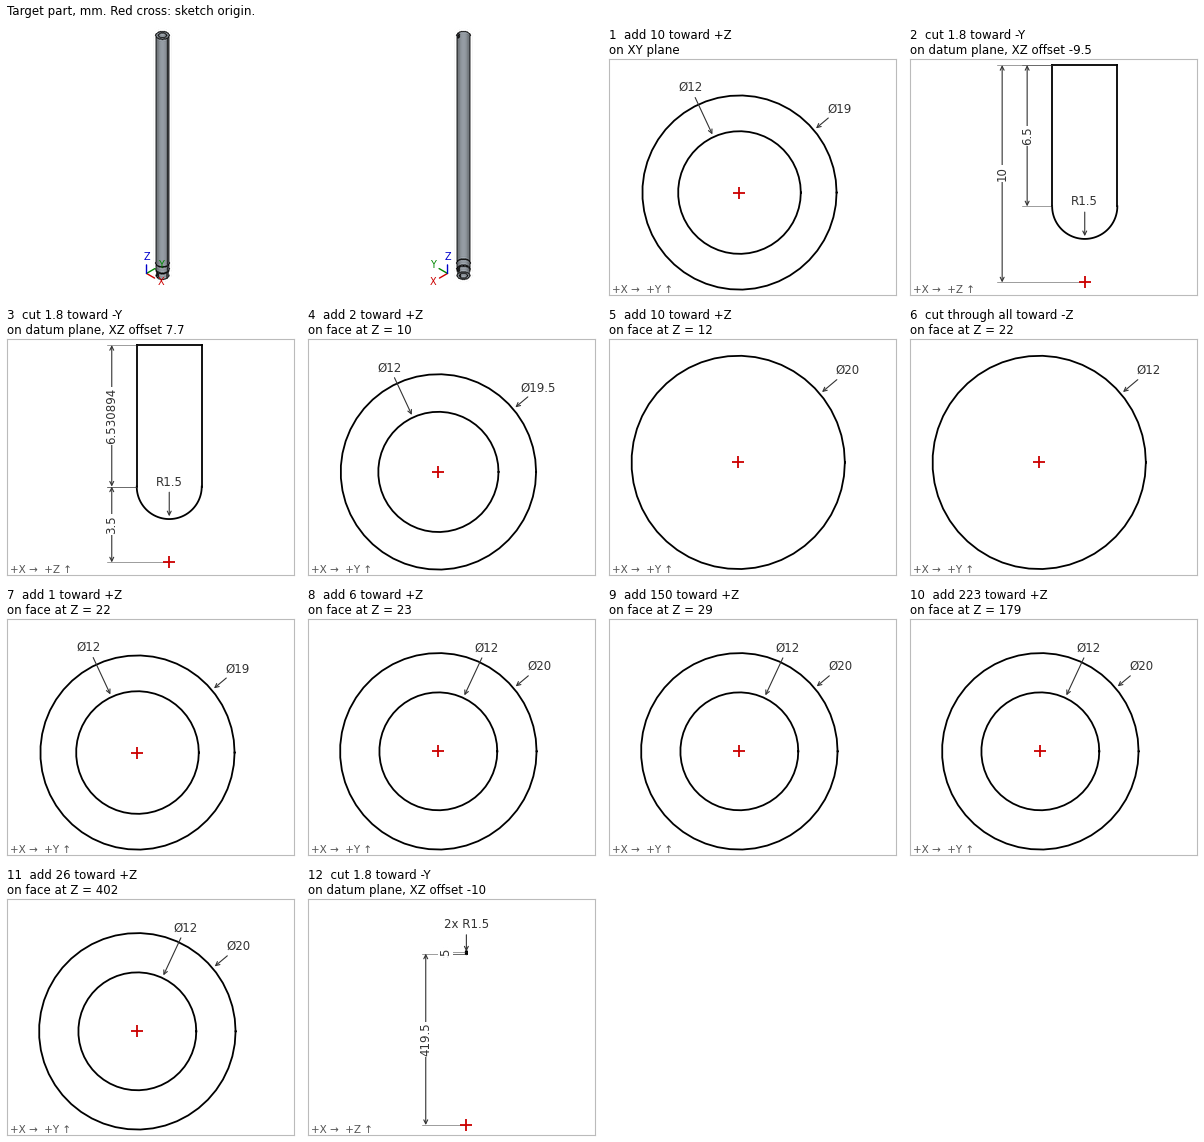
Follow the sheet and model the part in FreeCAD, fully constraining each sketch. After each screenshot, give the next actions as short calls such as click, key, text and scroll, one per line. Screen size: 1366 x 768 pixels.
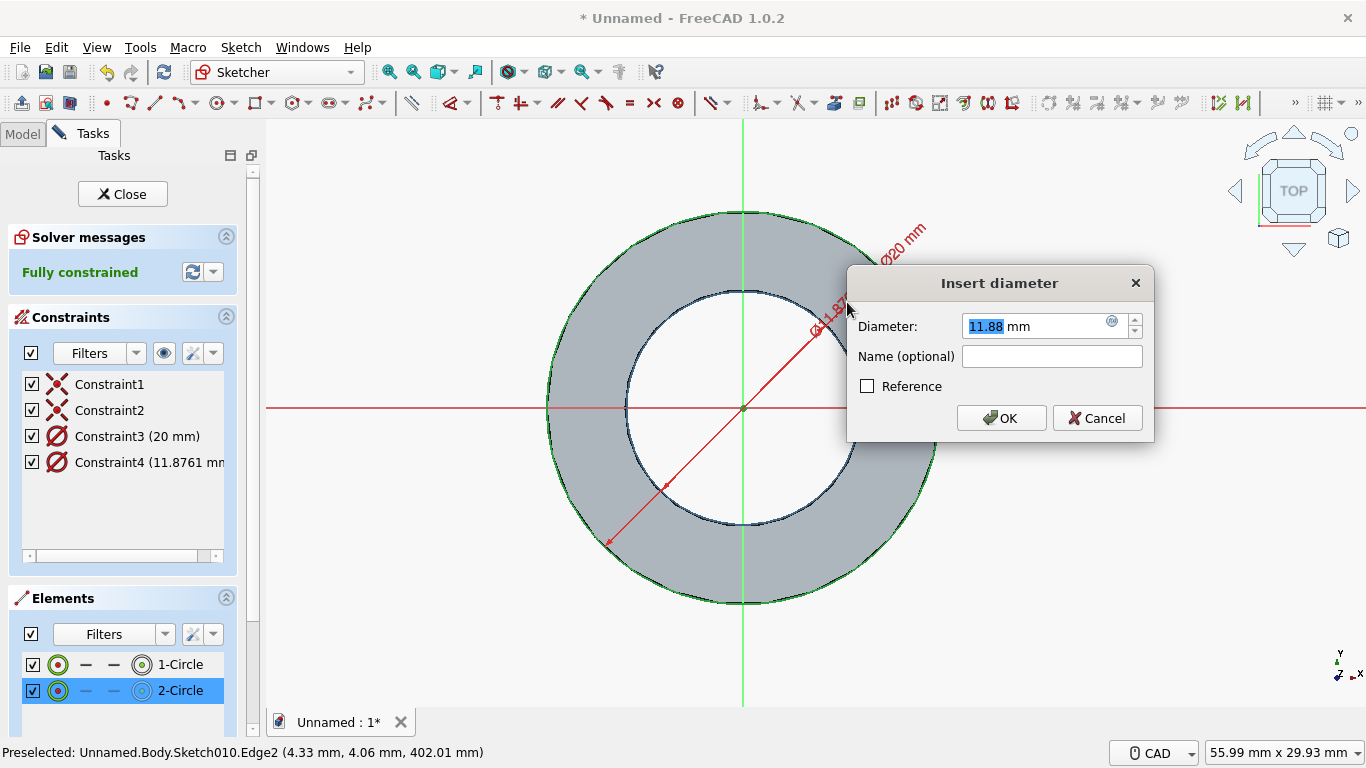
text(12)
key(Return)
key(Escape)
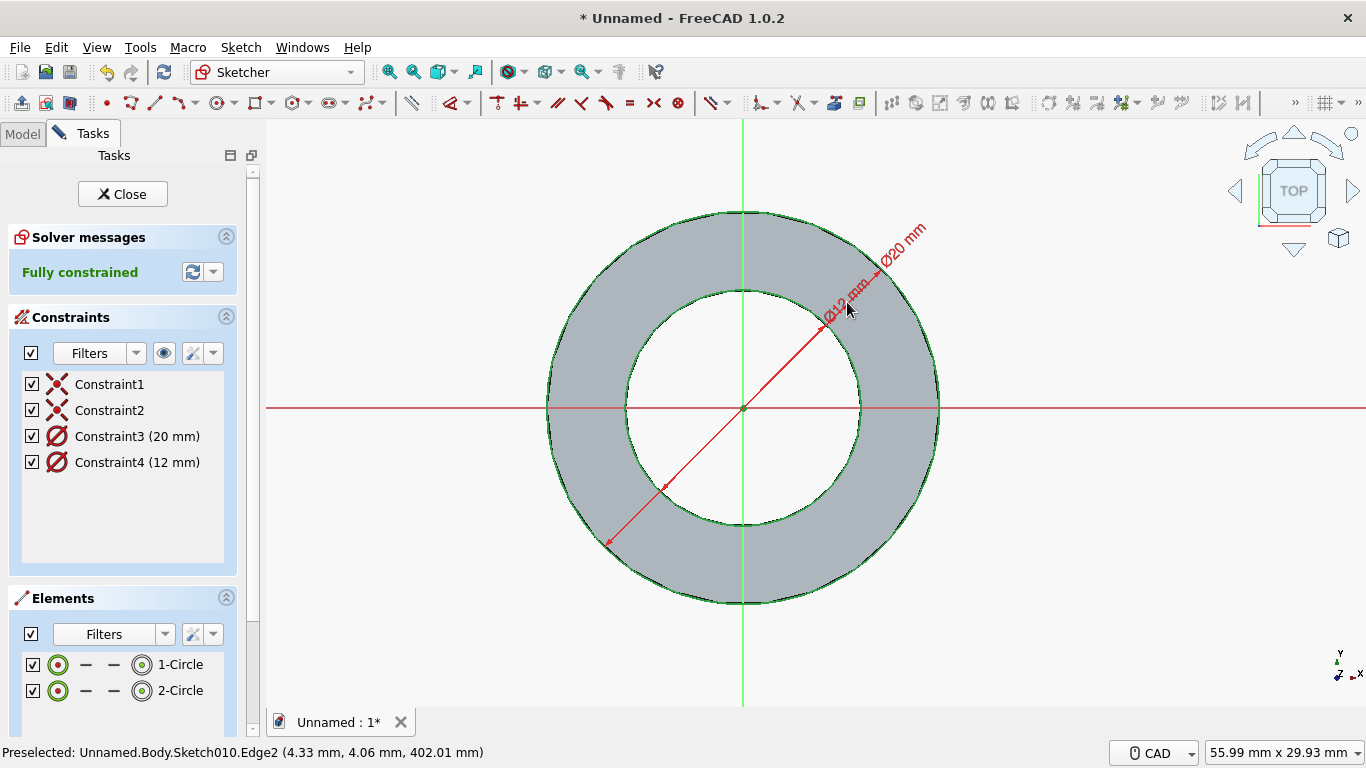
click(123, 194)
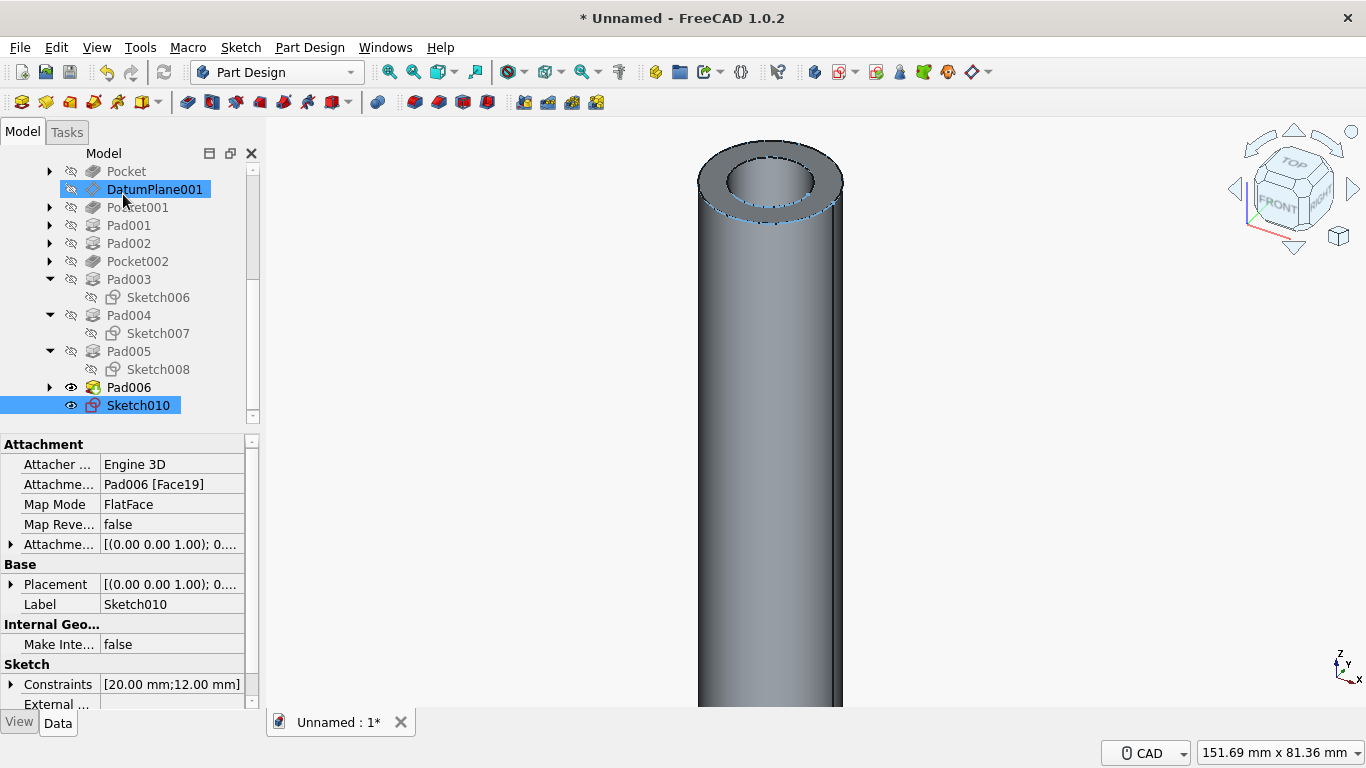
click(22, 102)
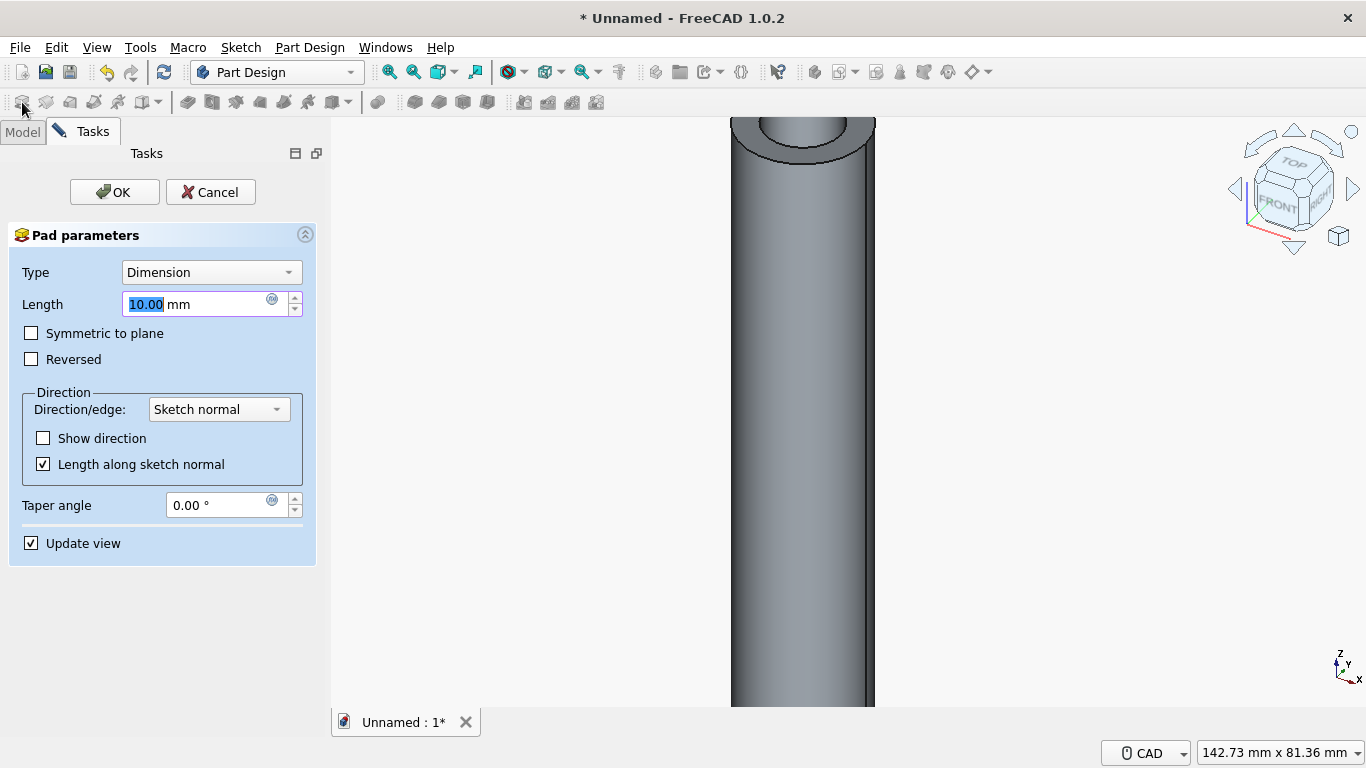
text(26)
key(Tab)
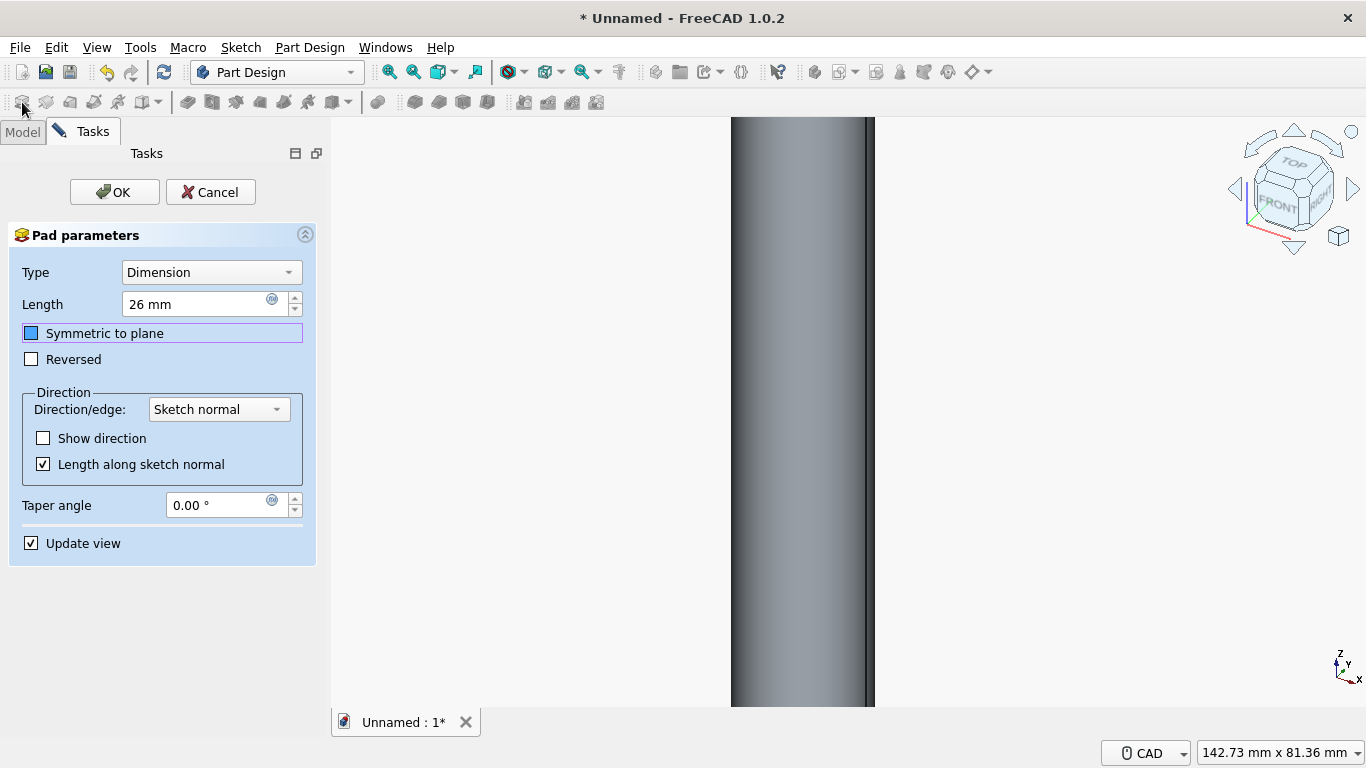
click(115, 192)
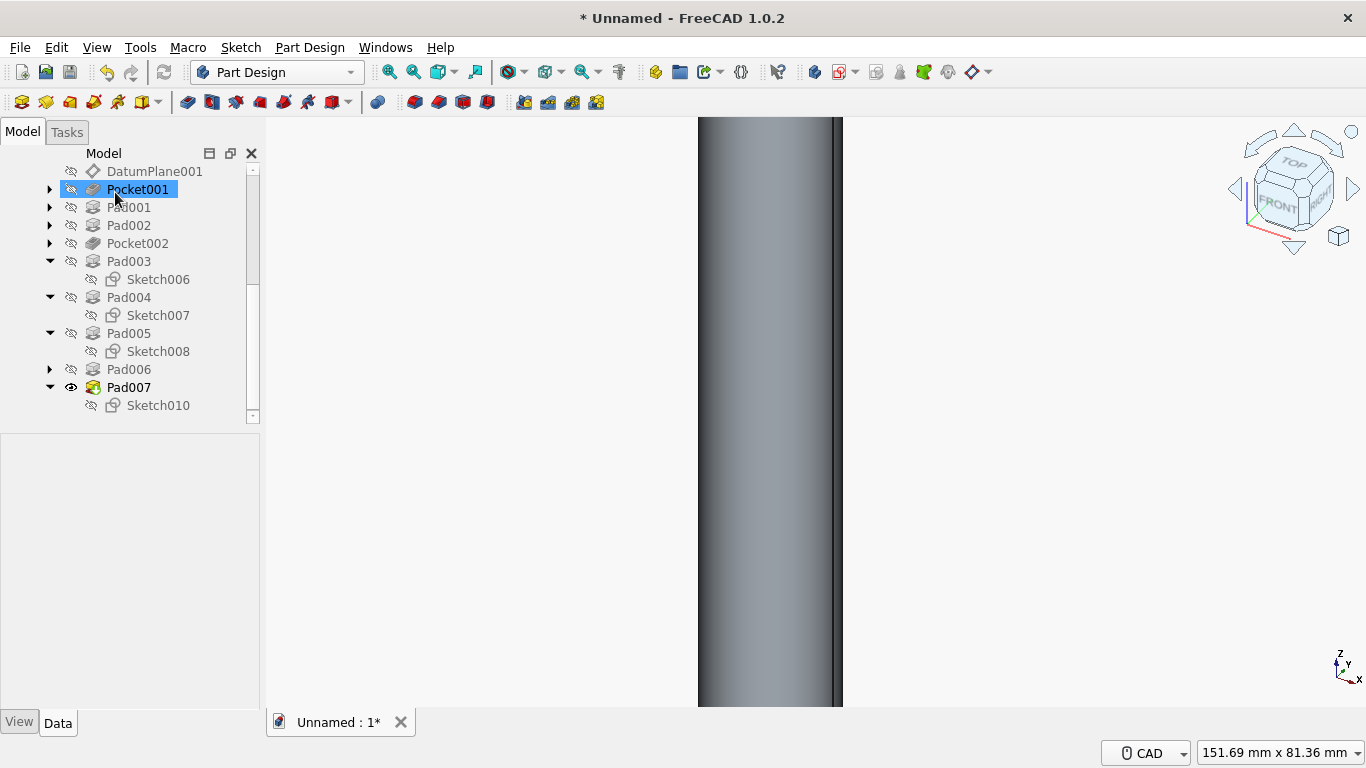
click(390, 72)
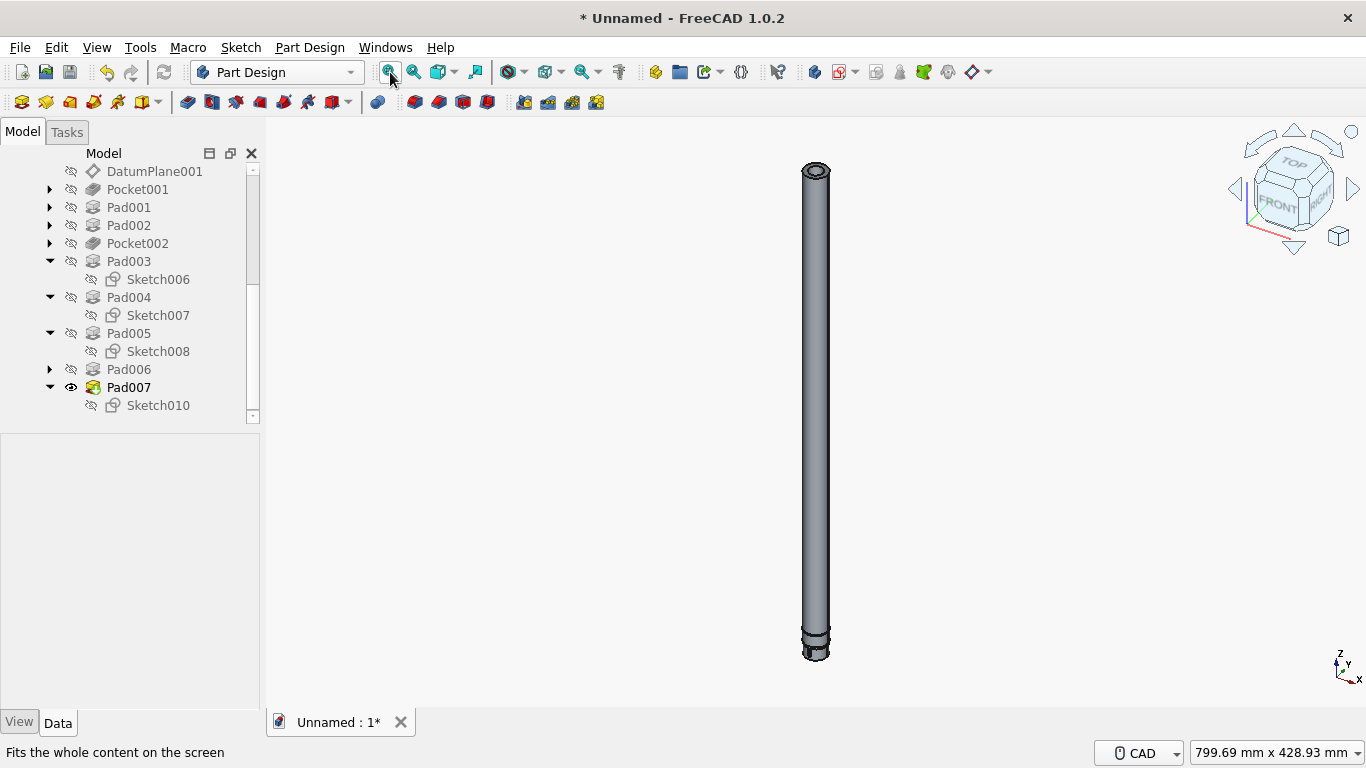
scroll(140, 293, down, 3)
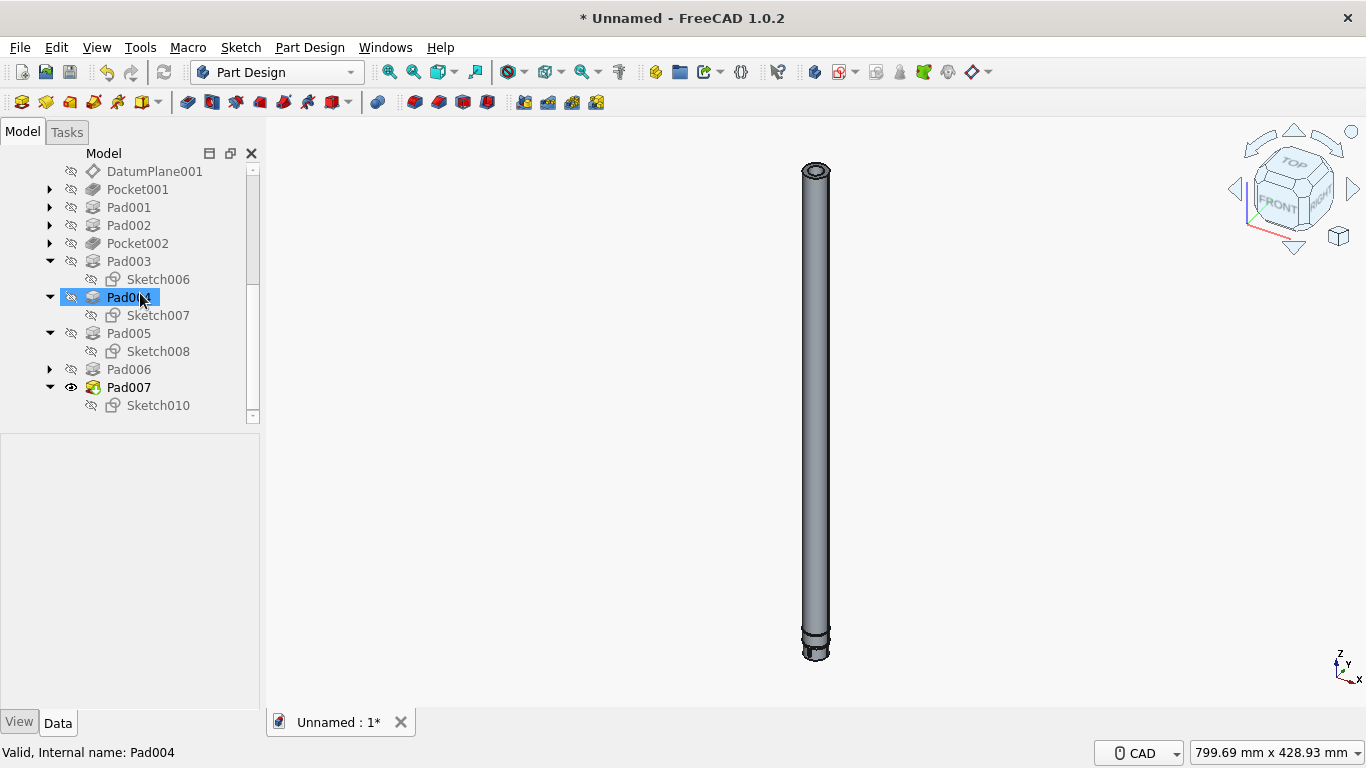
scroll(140, 293, up, 15)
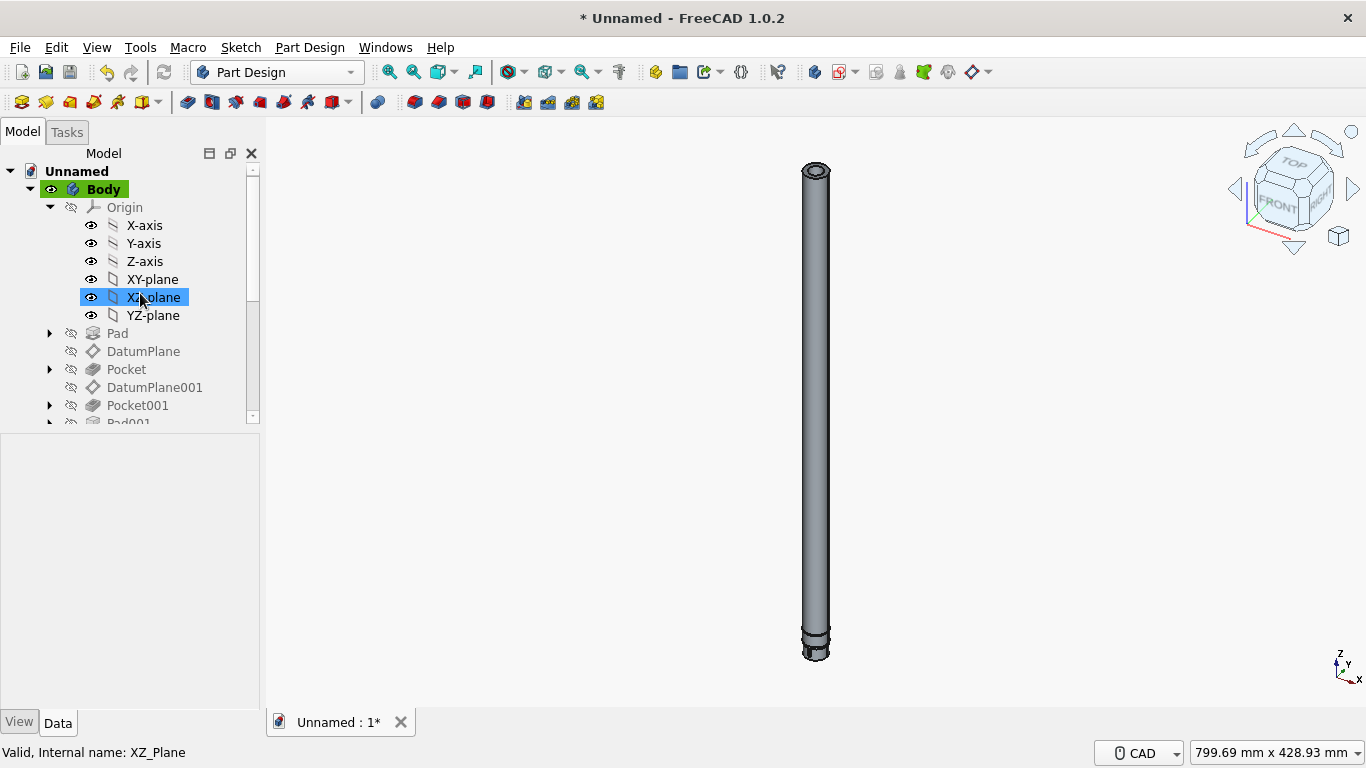
click(136, 297)